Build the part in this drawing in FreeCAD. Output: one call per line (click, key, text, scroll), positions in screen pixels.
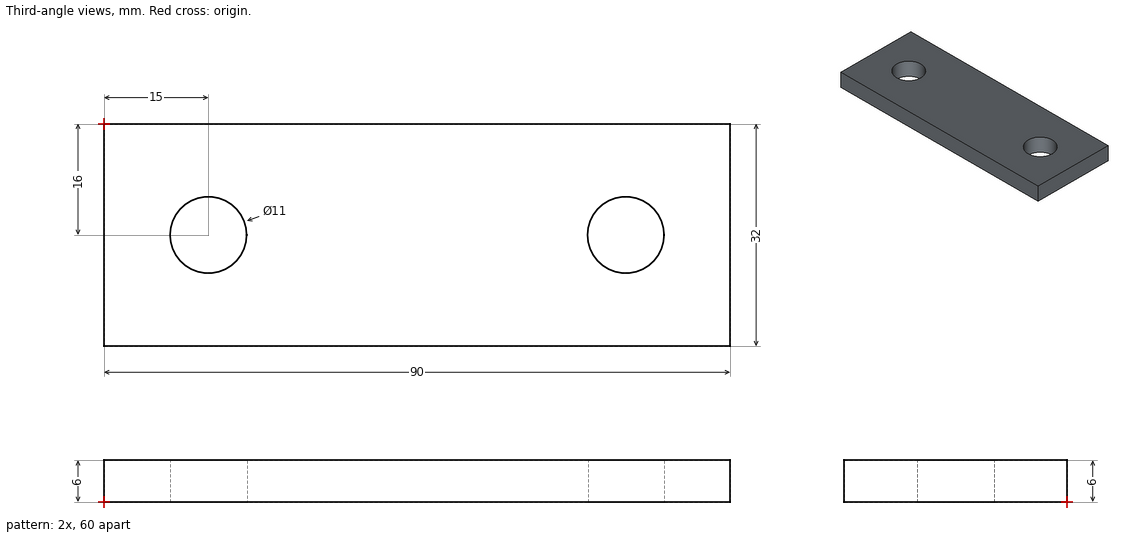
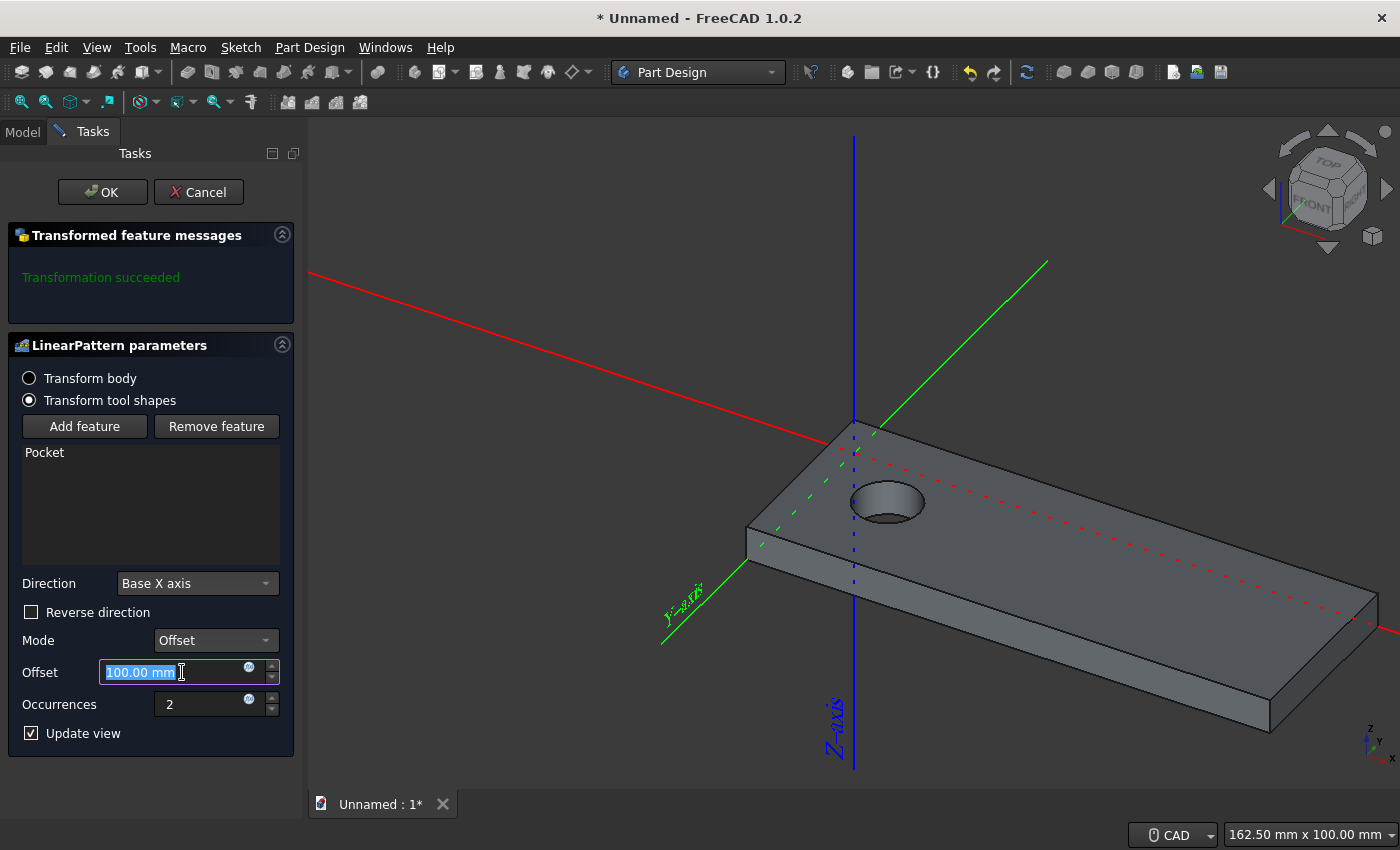
text(60)
key(Tab)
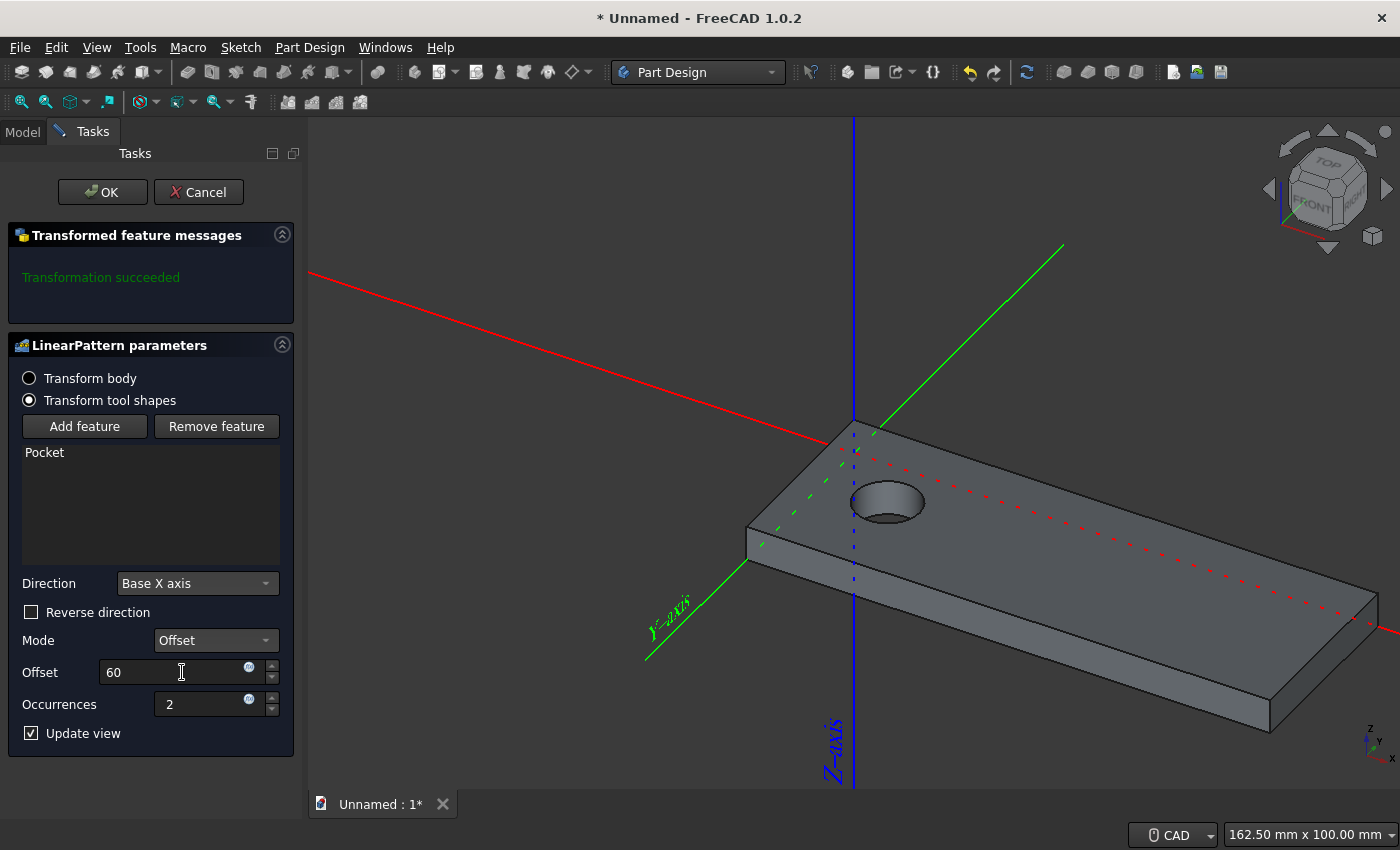
triple_click(209, 704)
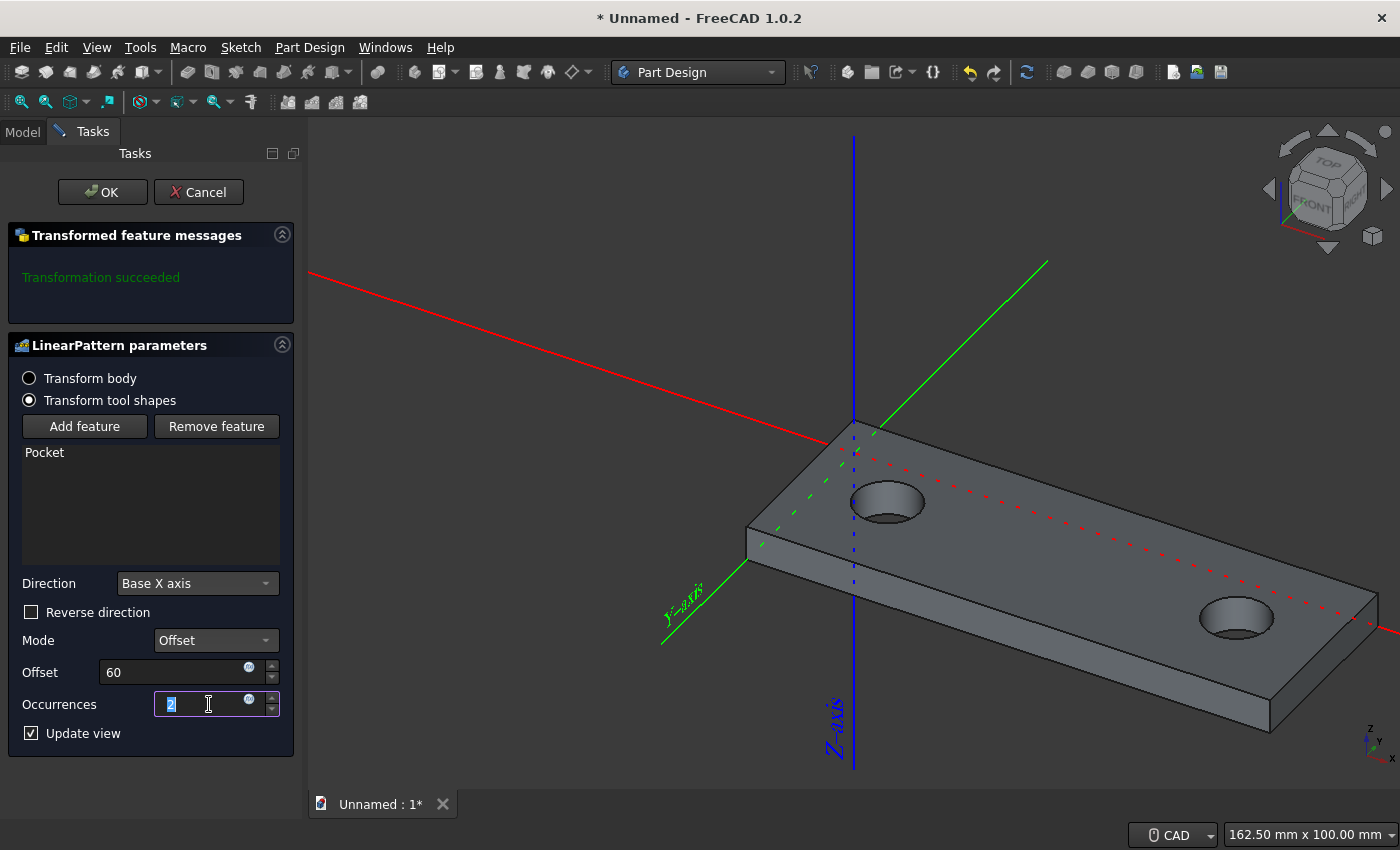
text(2)
key(Tab)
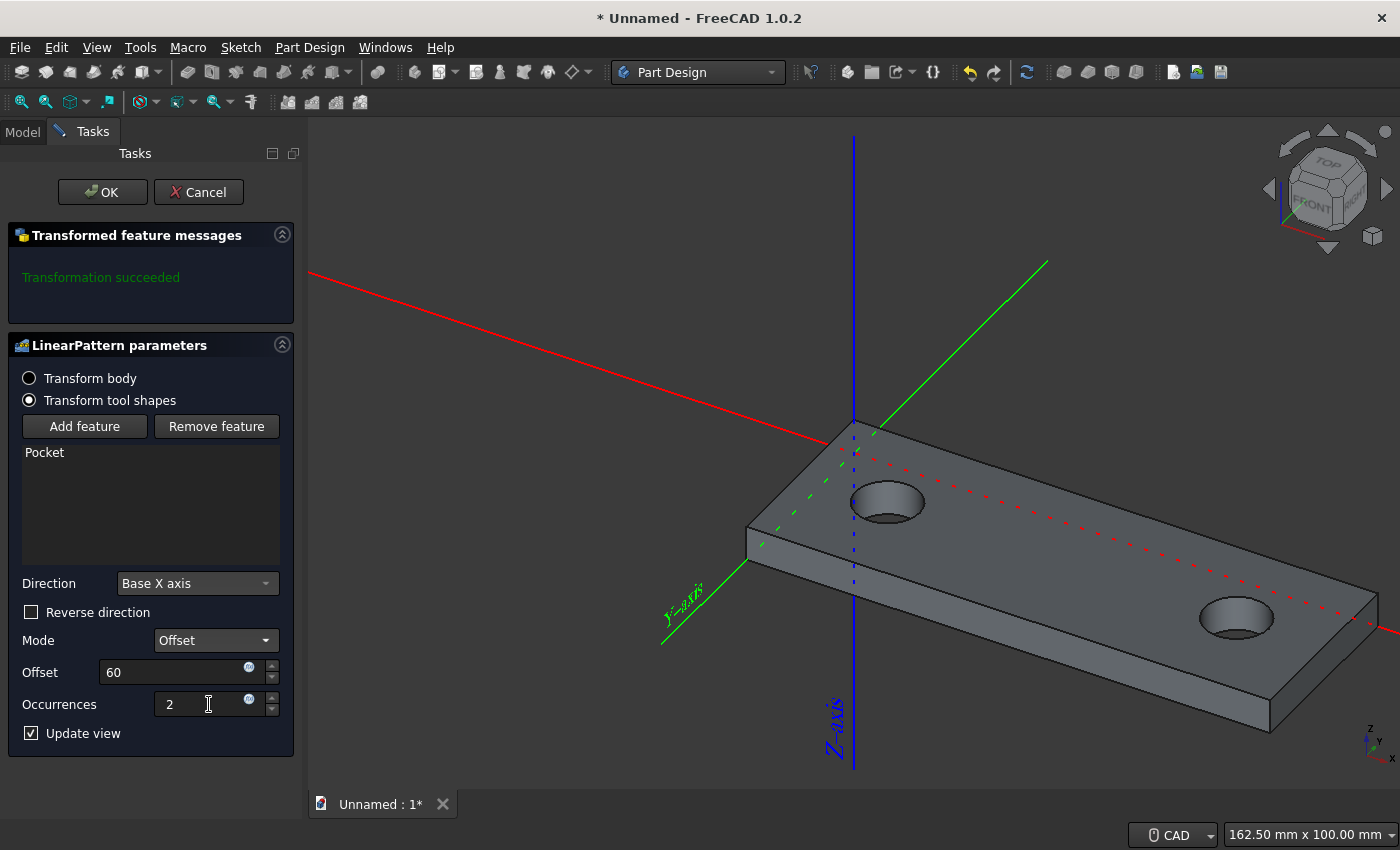
click(103, 192)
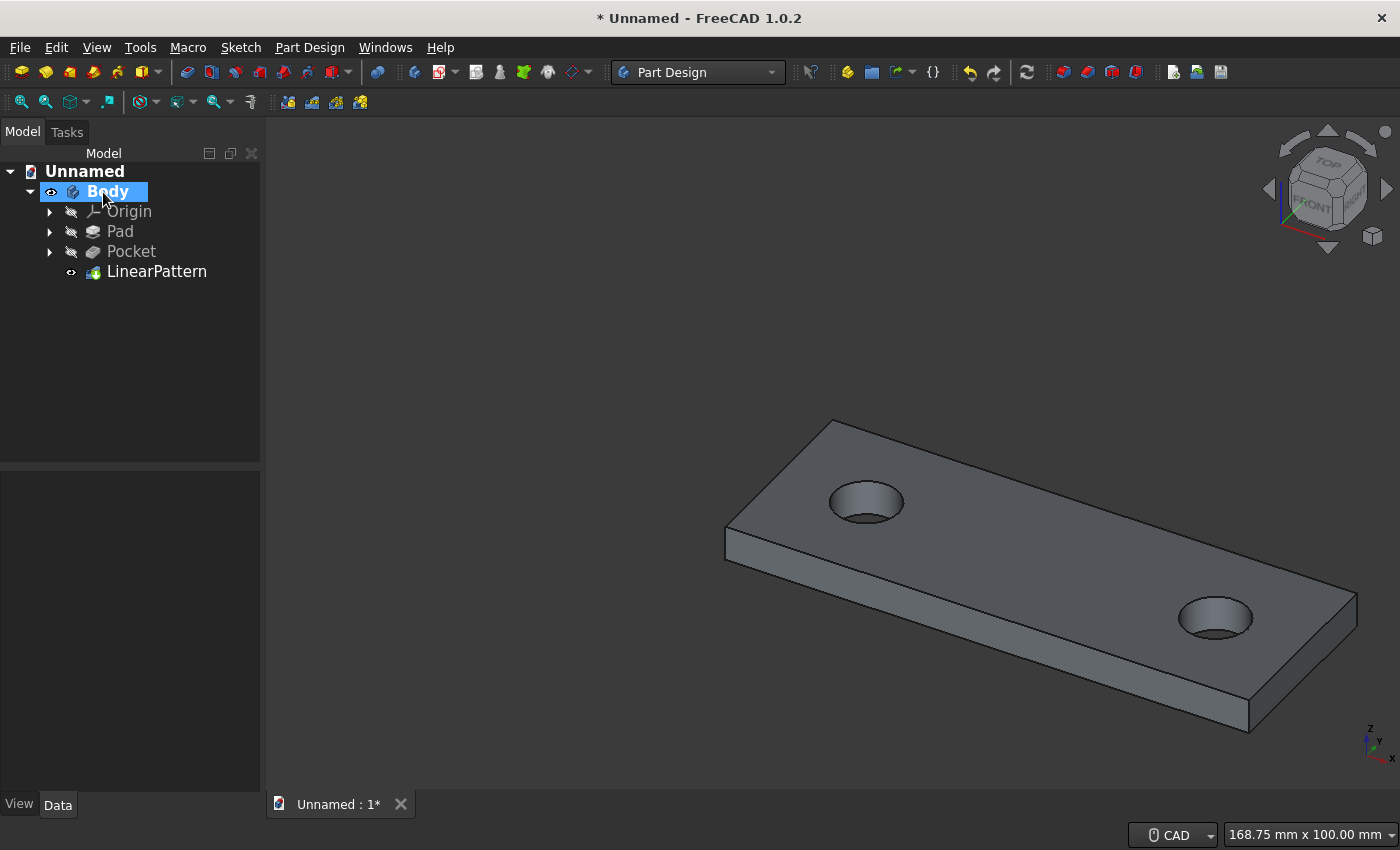
key(0)